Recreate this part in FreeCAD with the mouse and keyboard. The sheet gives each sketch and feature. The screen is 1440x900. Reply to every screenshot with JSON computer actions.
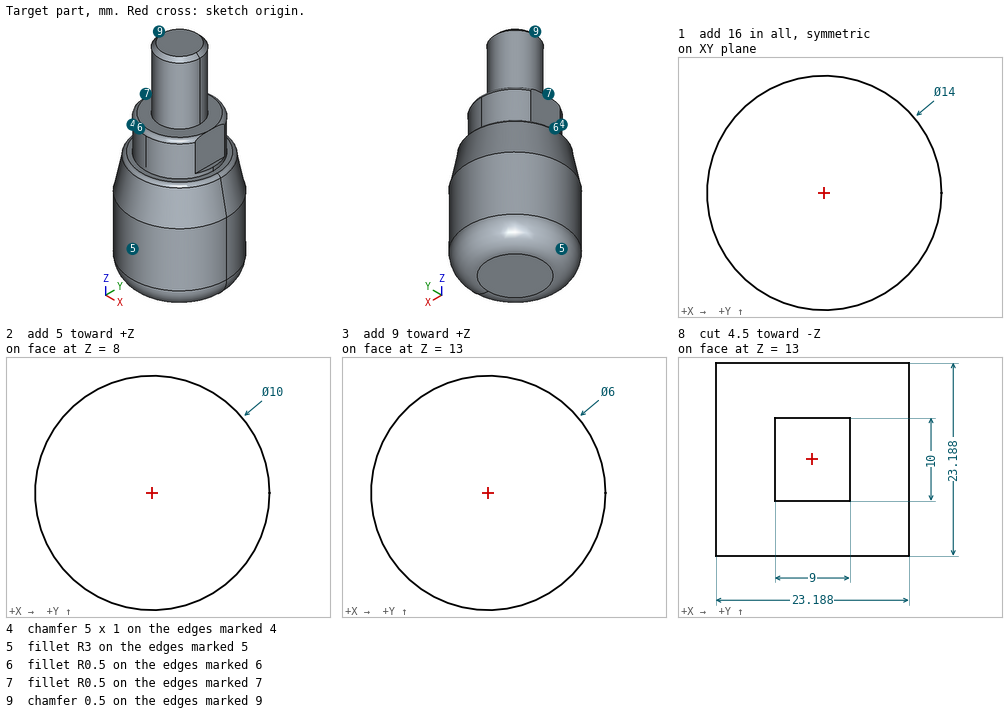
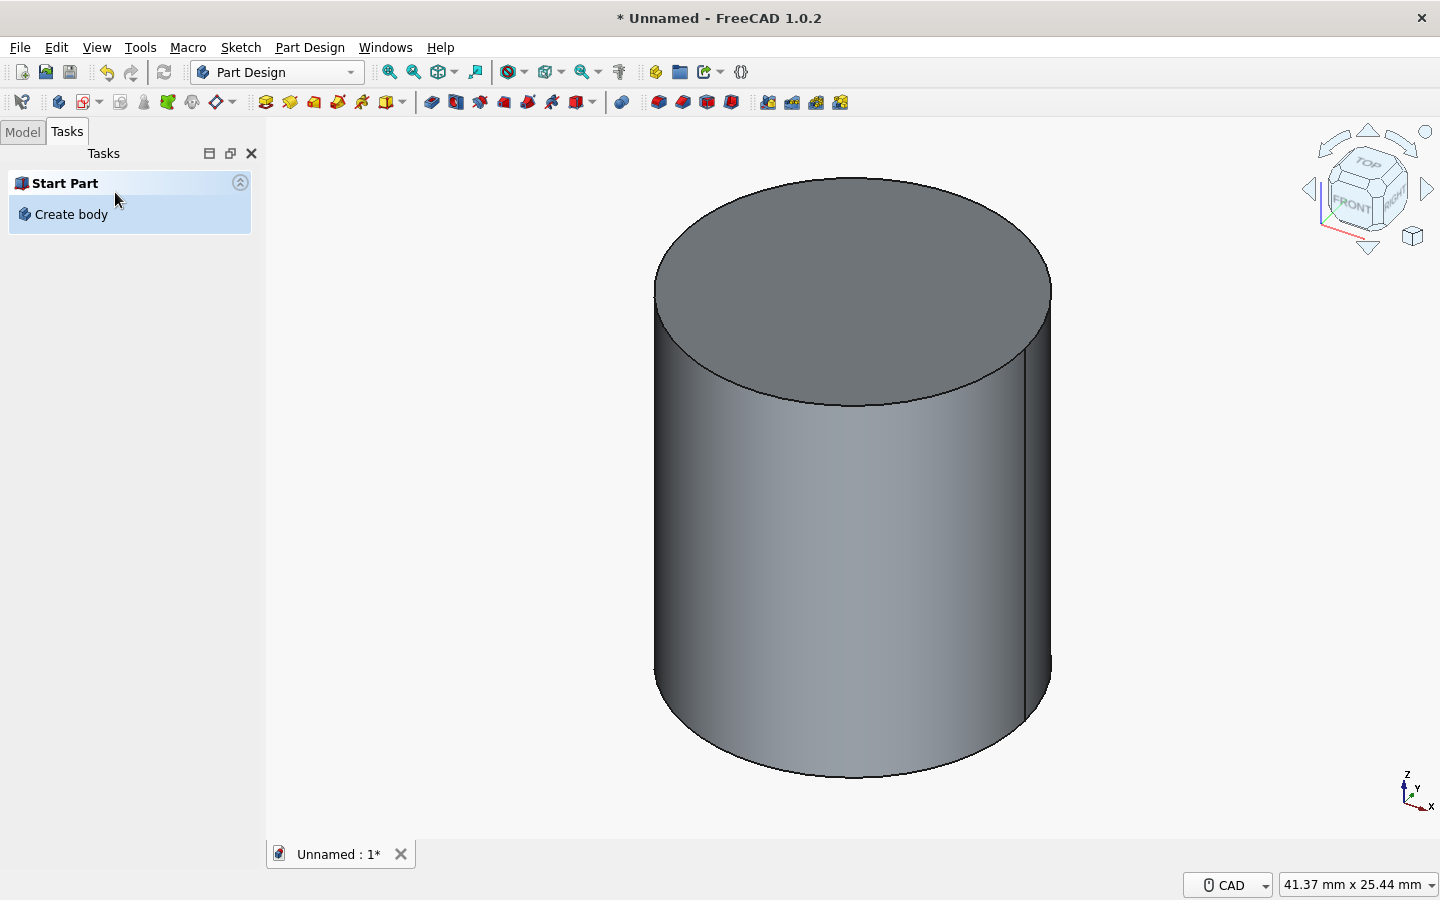
{"action": "left_click", "coordinate": [853, 291]}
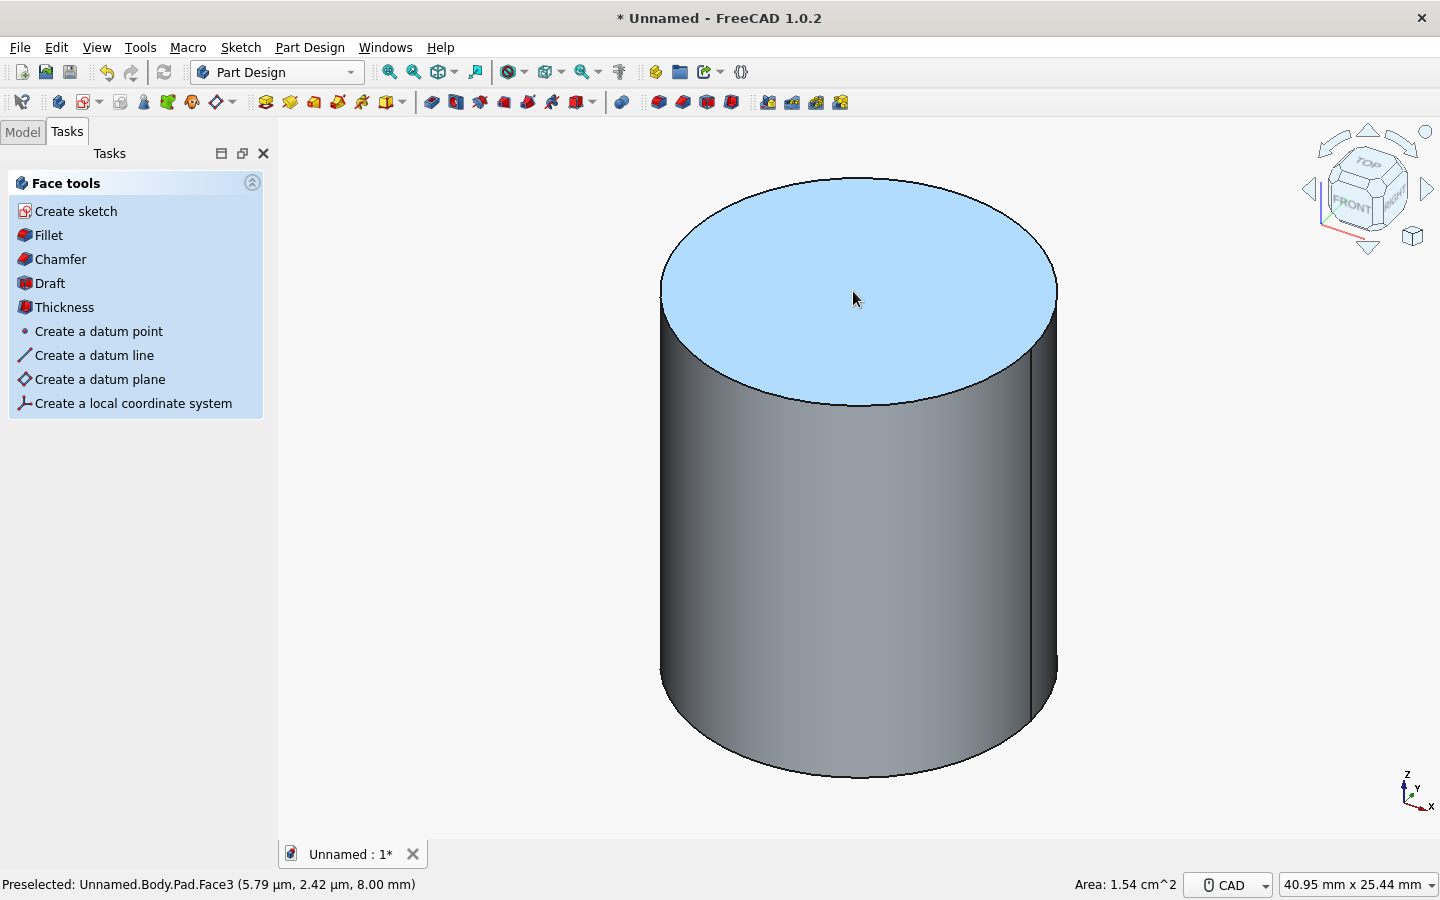
{"action": "left_click", "coordinate": [84, 102]}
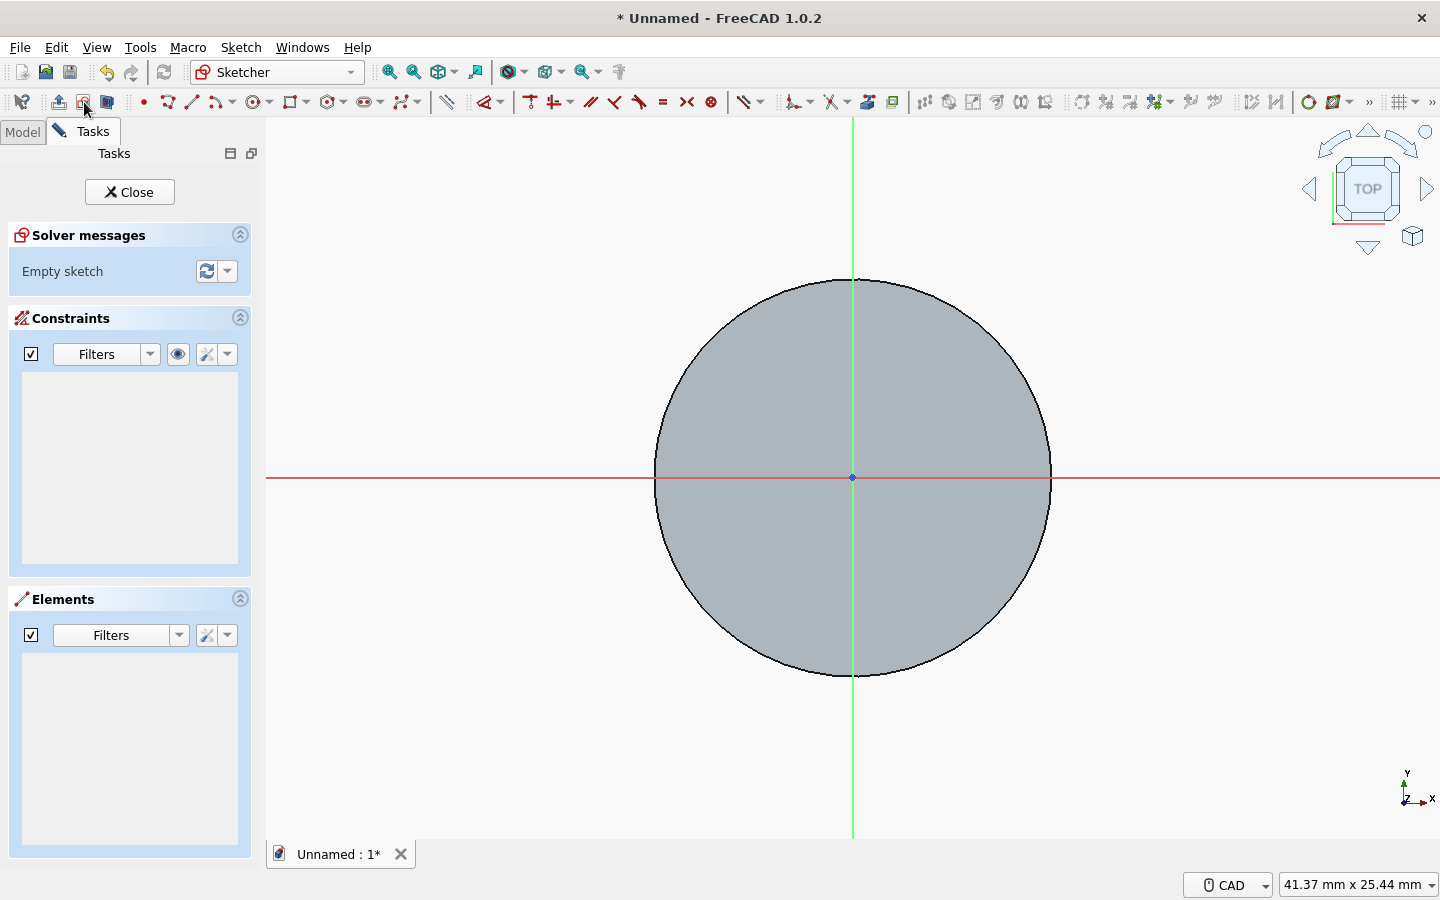
{"action": "scroll", "coordinate": [936, 478], "scroll_direction": "up", "scroll_amount": 3}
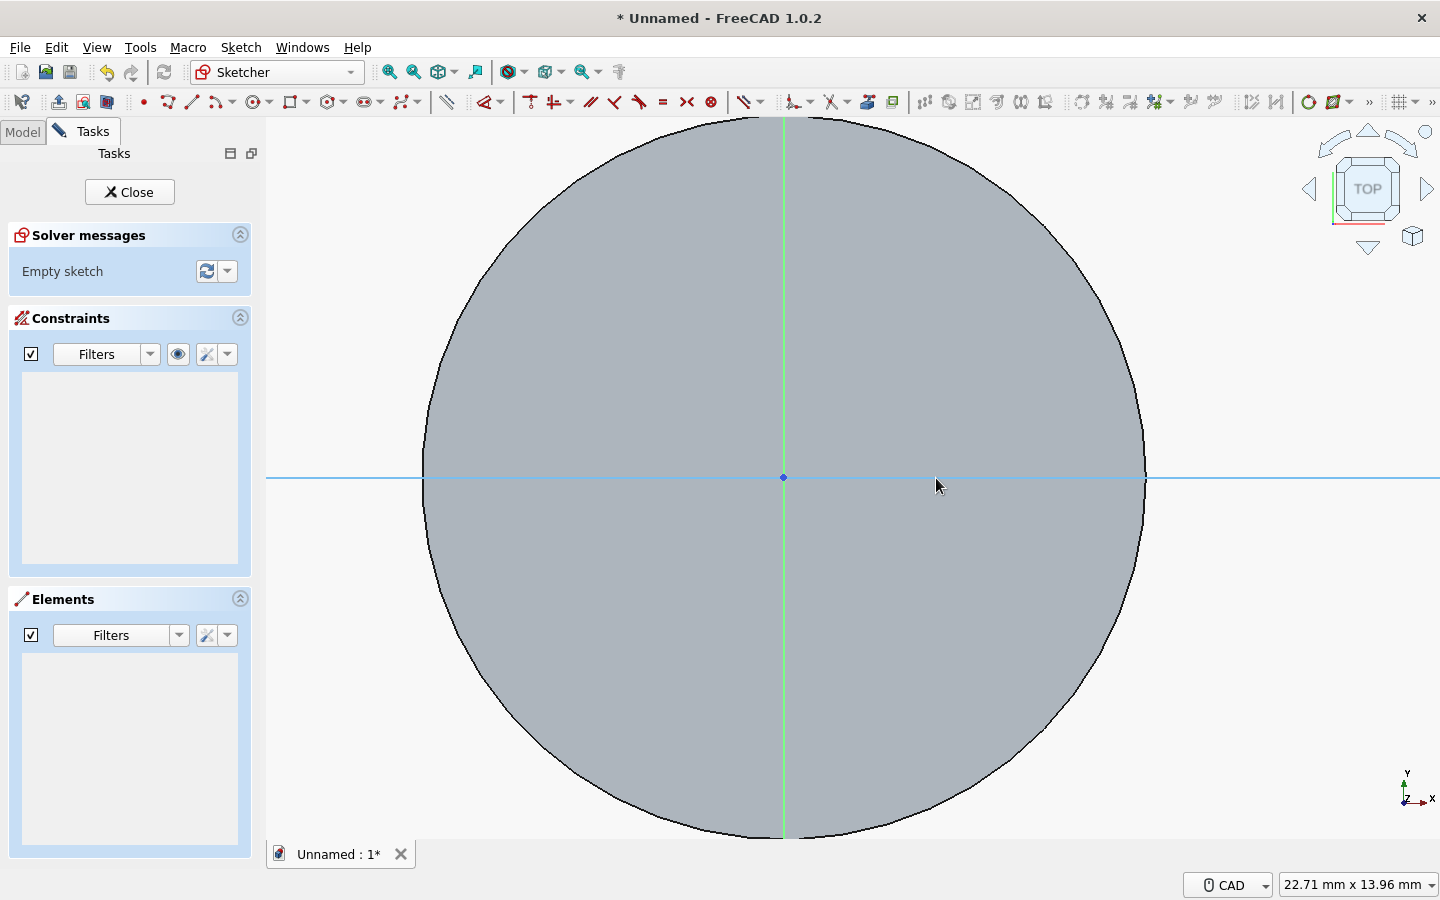
{"action": "key", "text": "g c"}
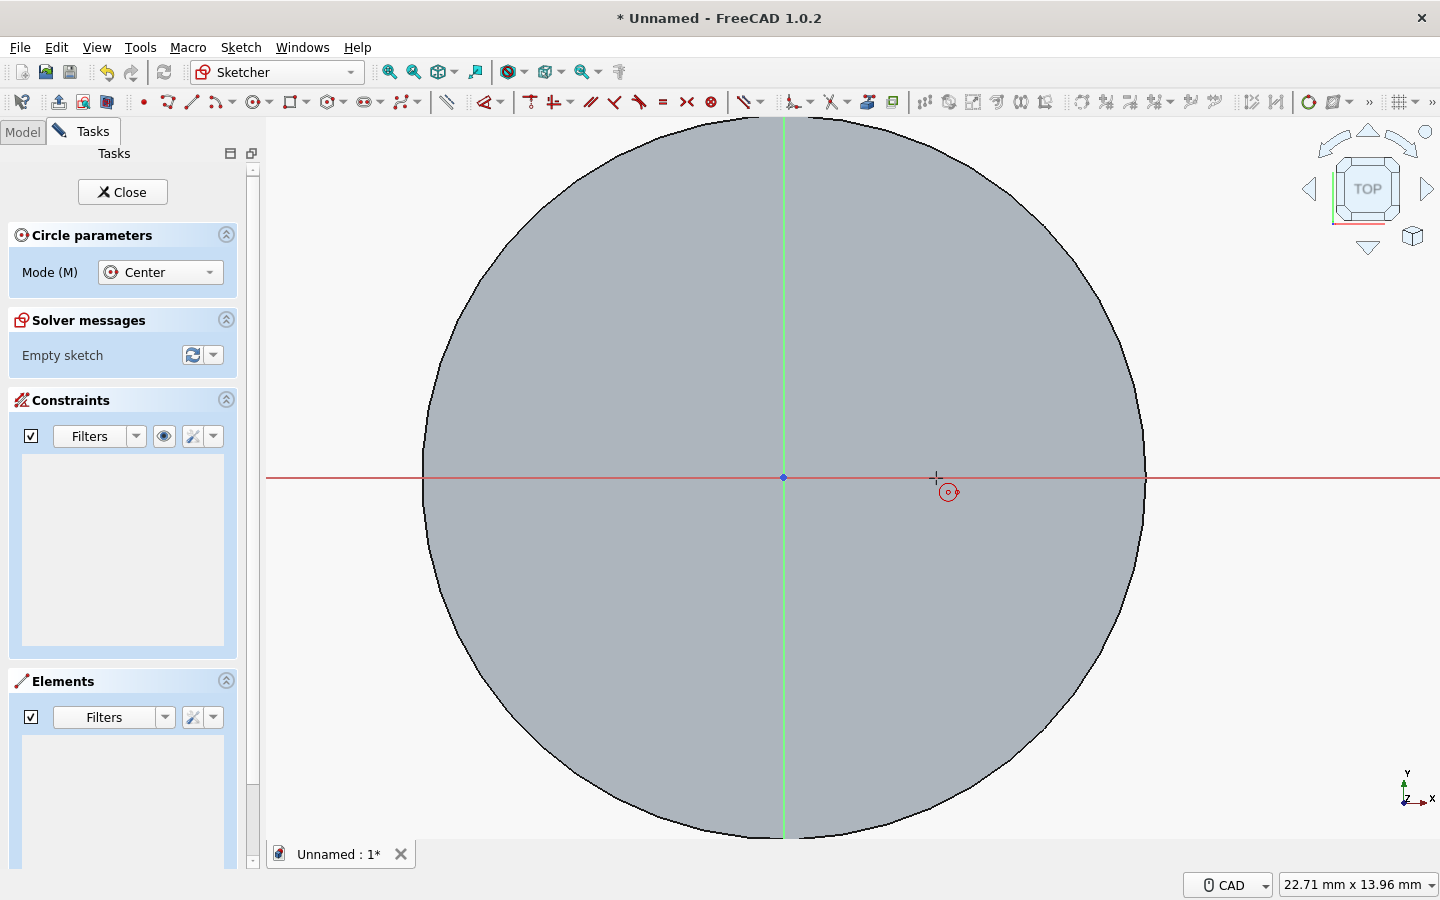
{"action": "left_click", "coordinate": [784, 478]}
{"action": "left_click", "coordinate": [967, 295]}
{"action": "key", "text": "Escape"}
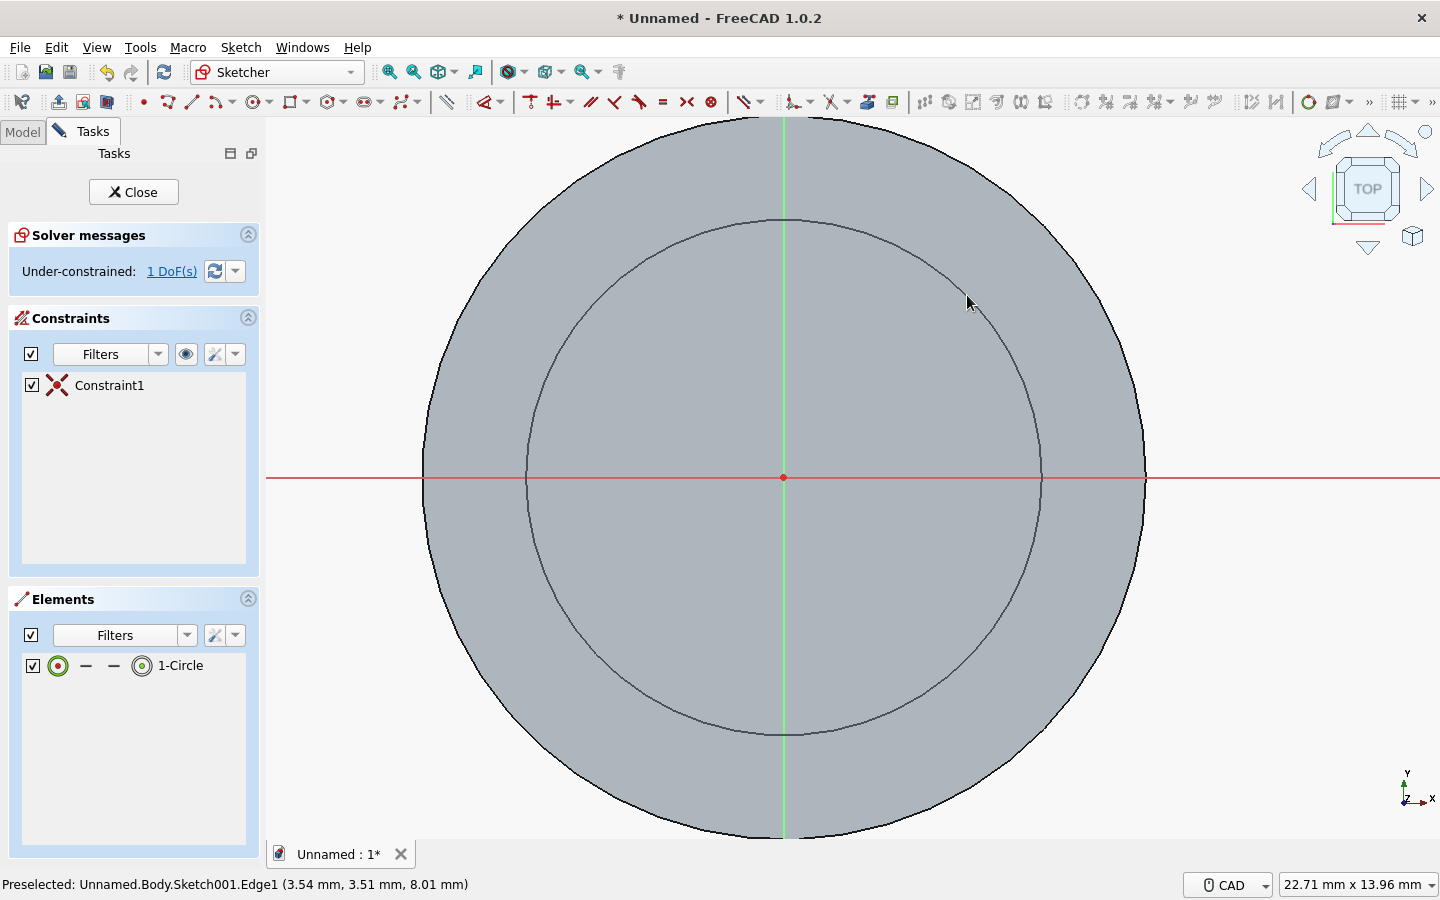
{"action": "left_click", "coordinate": [966, 295]}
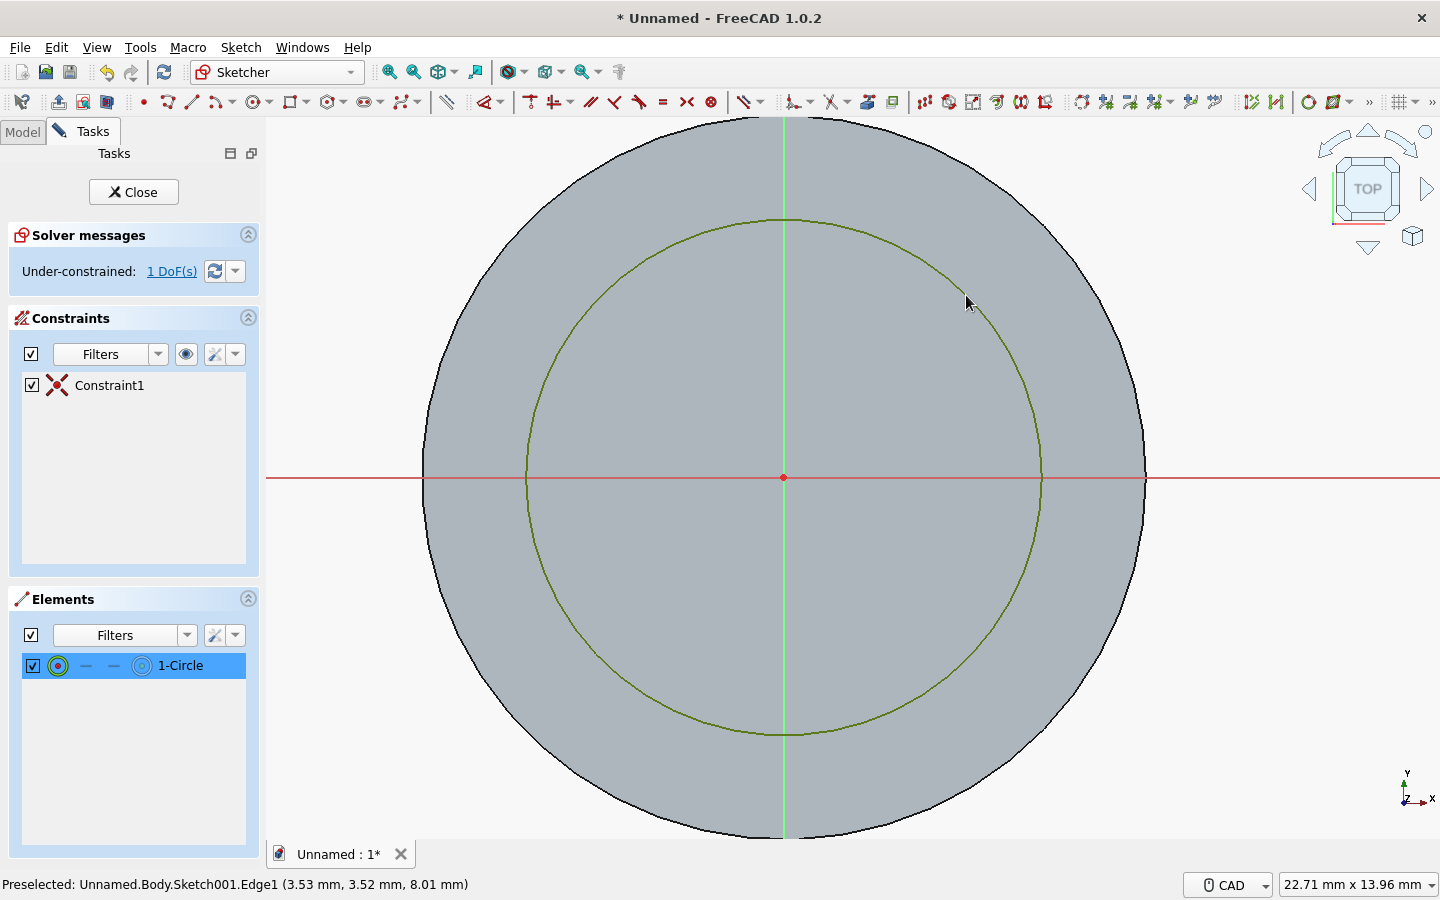
{"action": "key", "text": "k o"}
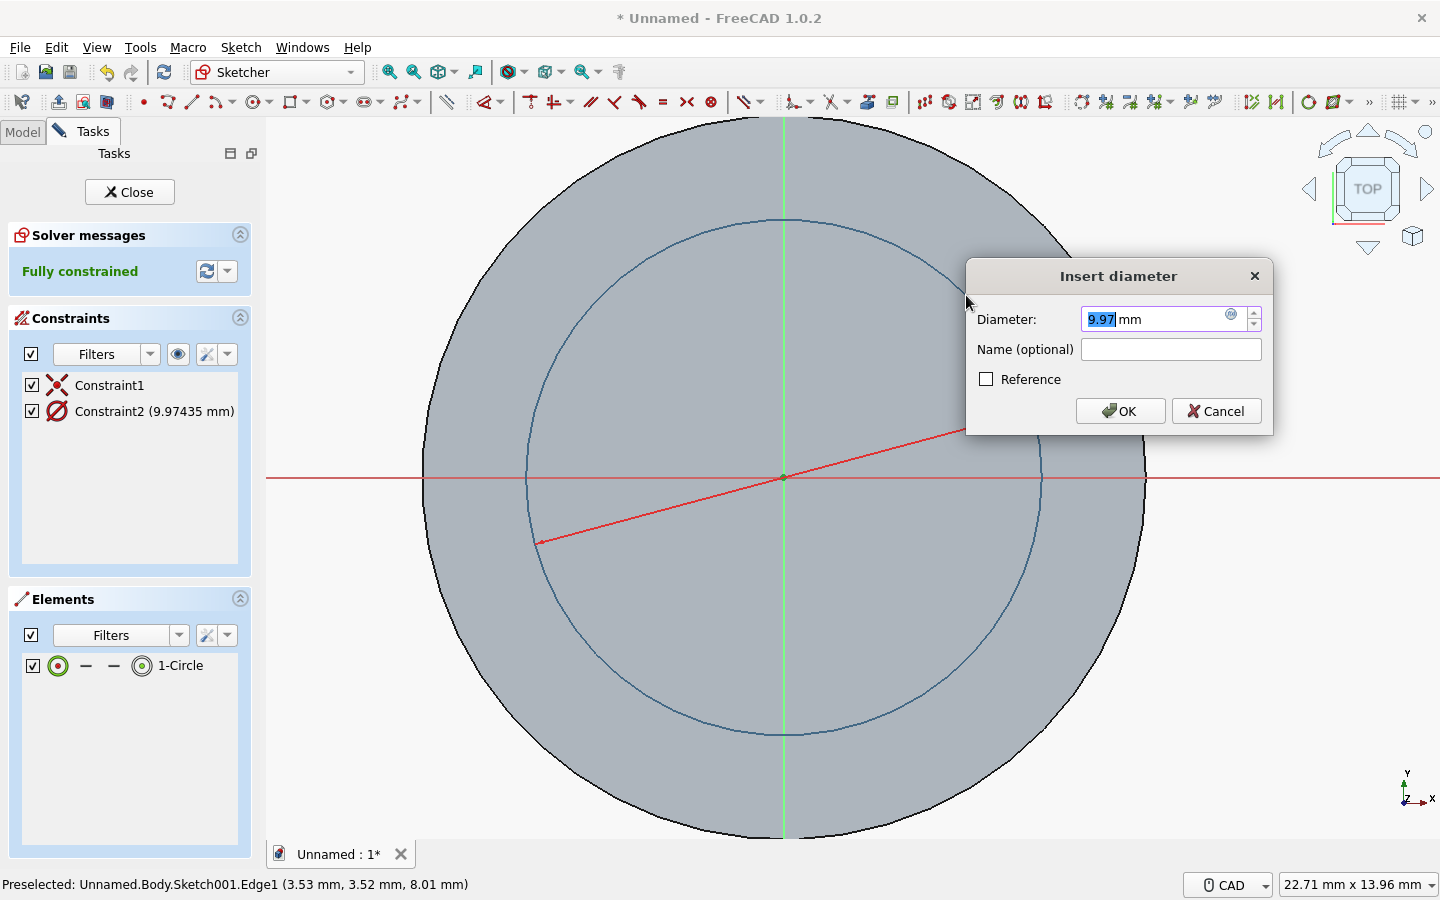
{"action": "type", "text": "10"}
{"action": "key", "text": "Return"}